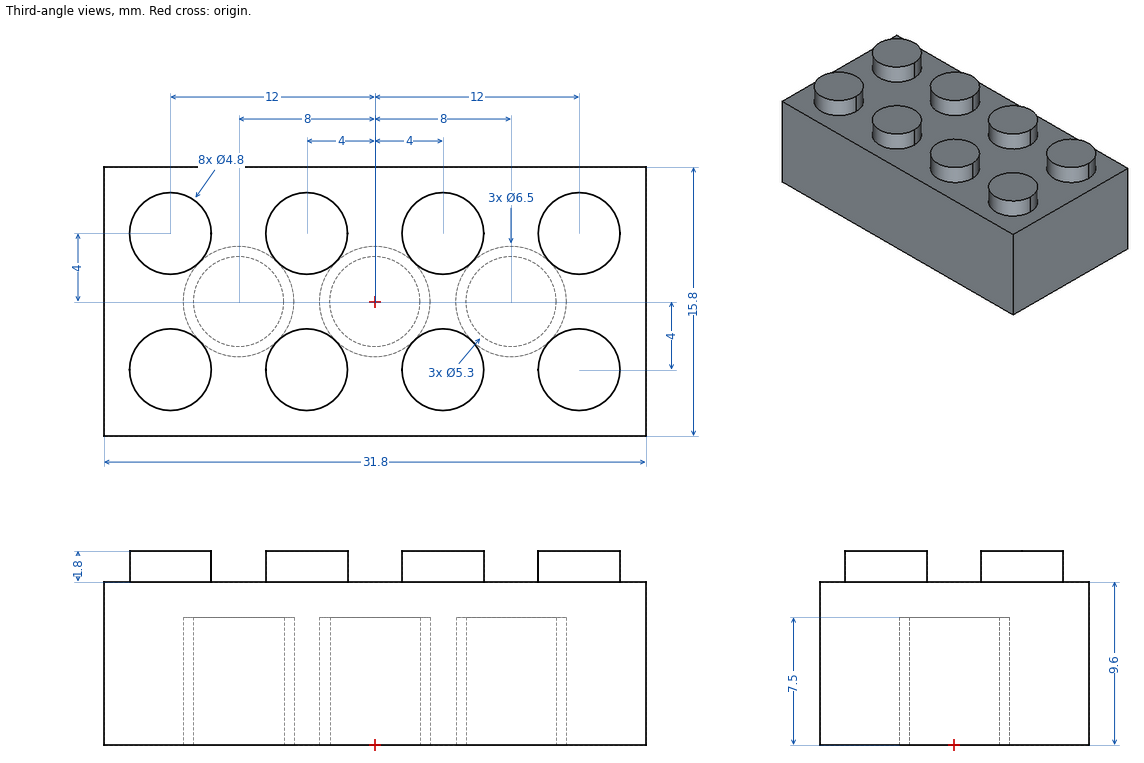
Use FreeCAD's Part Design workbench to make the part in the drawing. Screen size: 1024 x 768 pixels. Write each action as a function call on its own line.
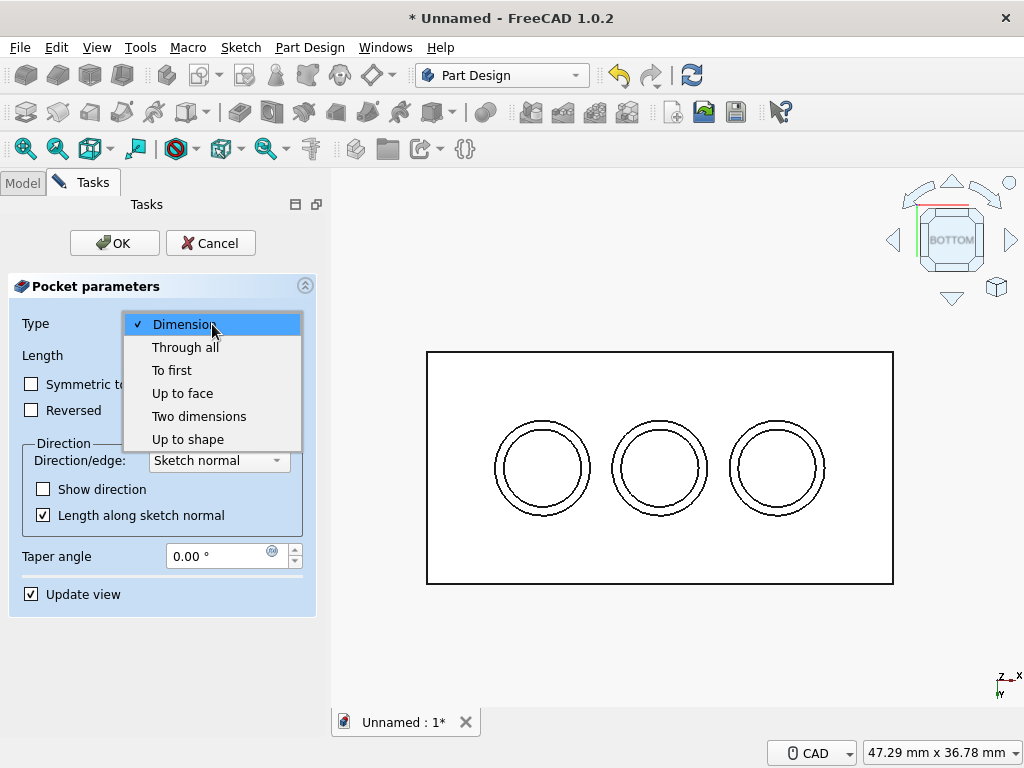
click(212, 416)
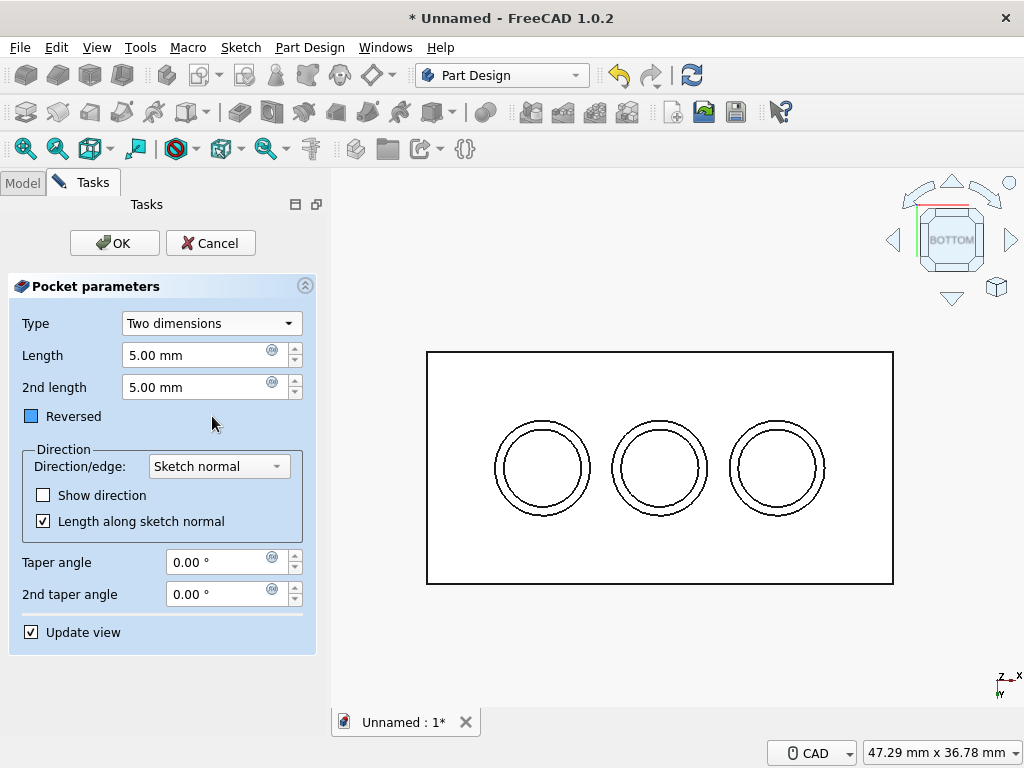
triple_click(204, 355)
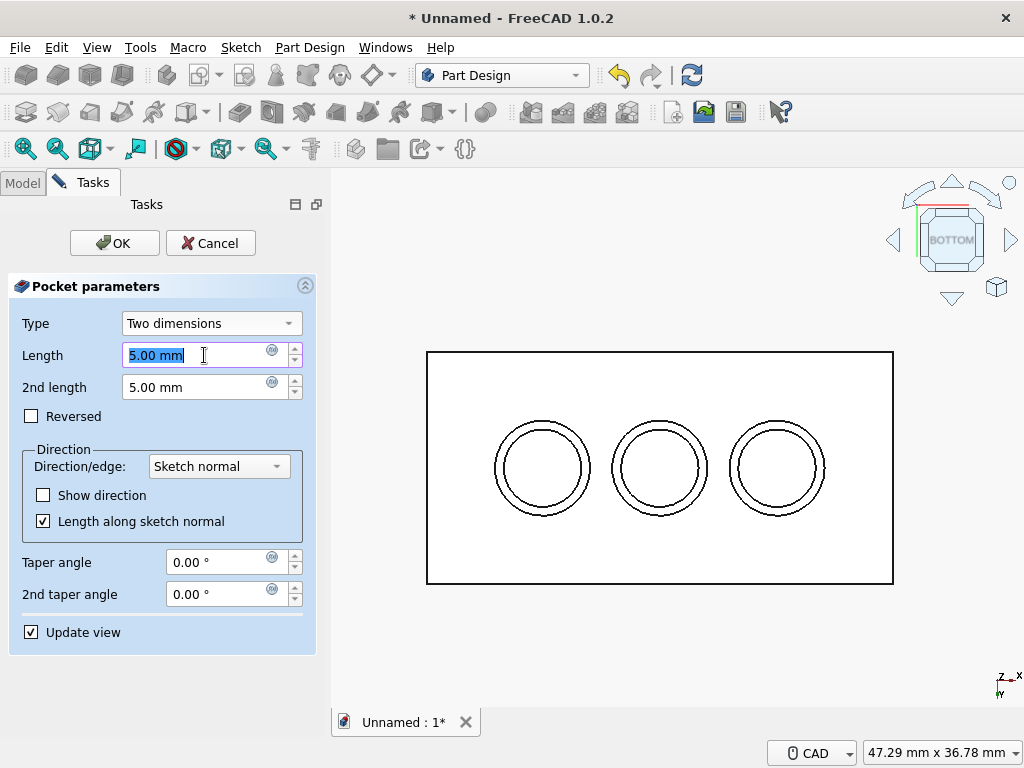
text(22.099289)
key(Tab)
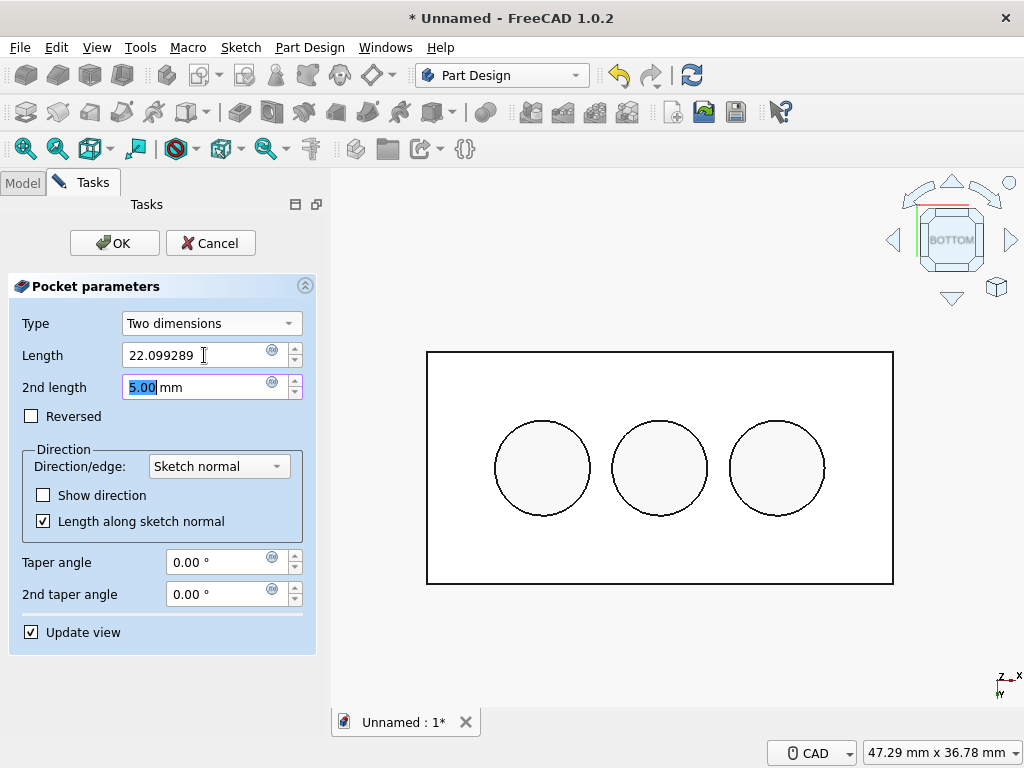
text(7.5)
key(Tab)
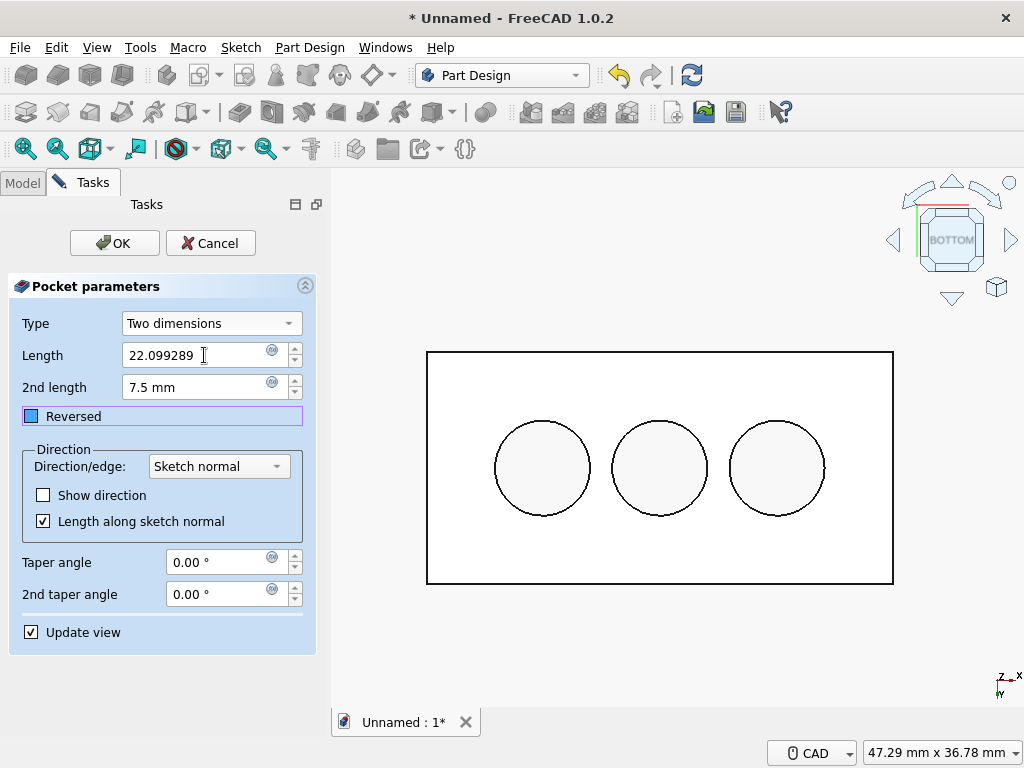
click(30, 416)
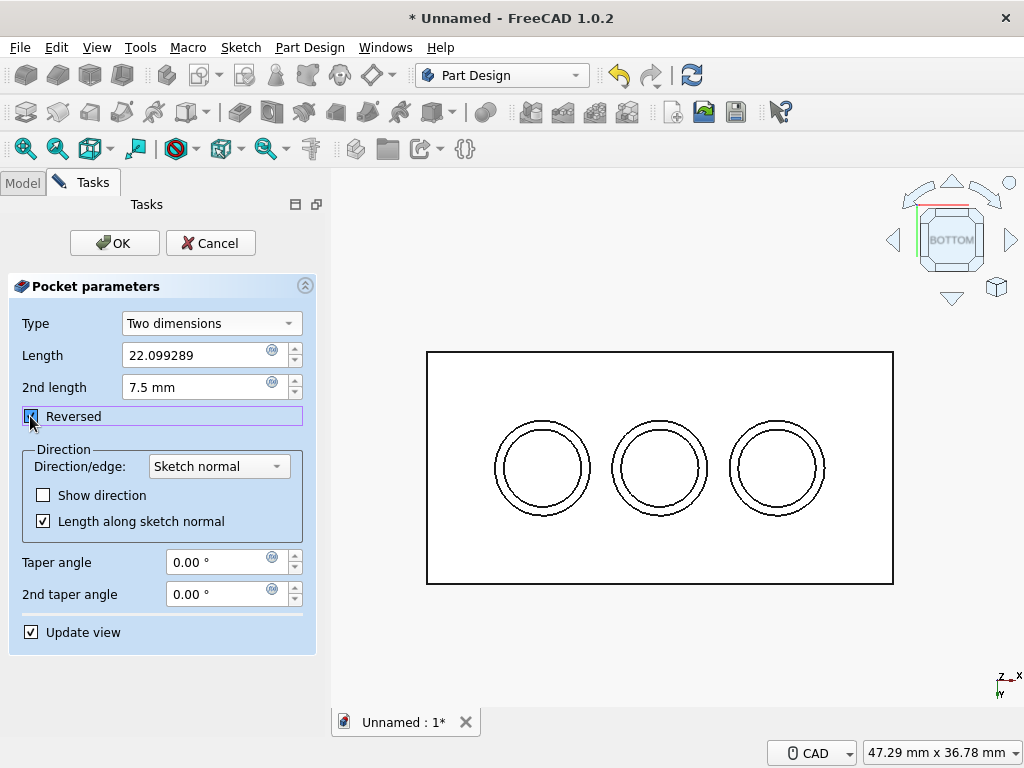
click(115, 243)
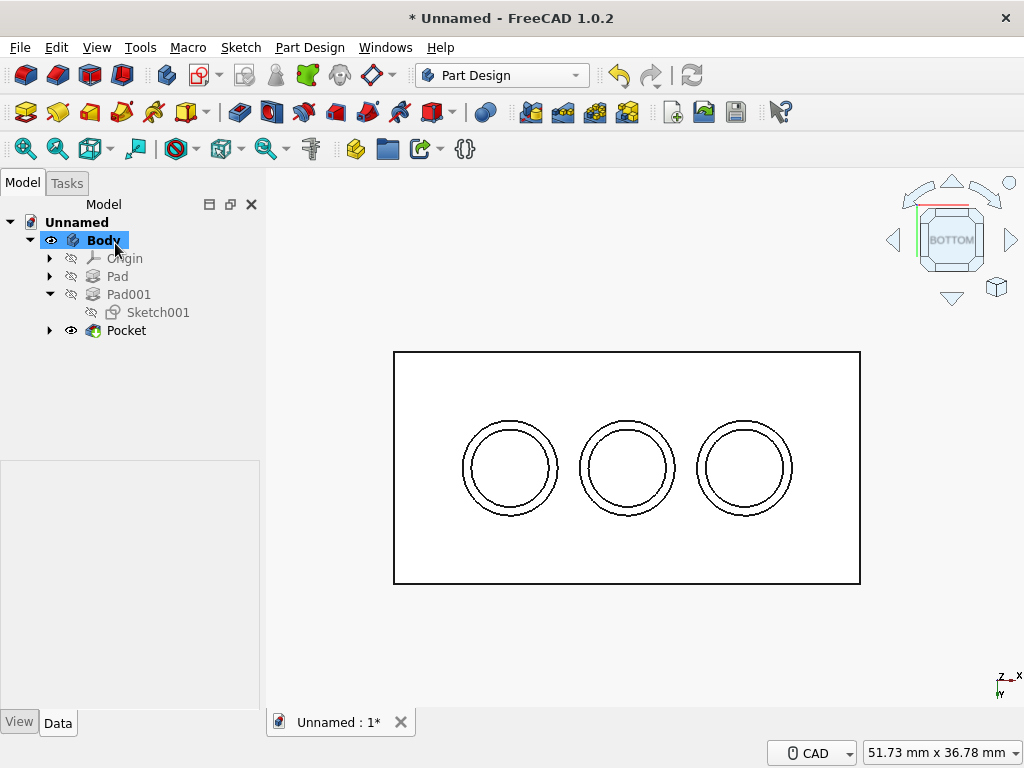
key(0)